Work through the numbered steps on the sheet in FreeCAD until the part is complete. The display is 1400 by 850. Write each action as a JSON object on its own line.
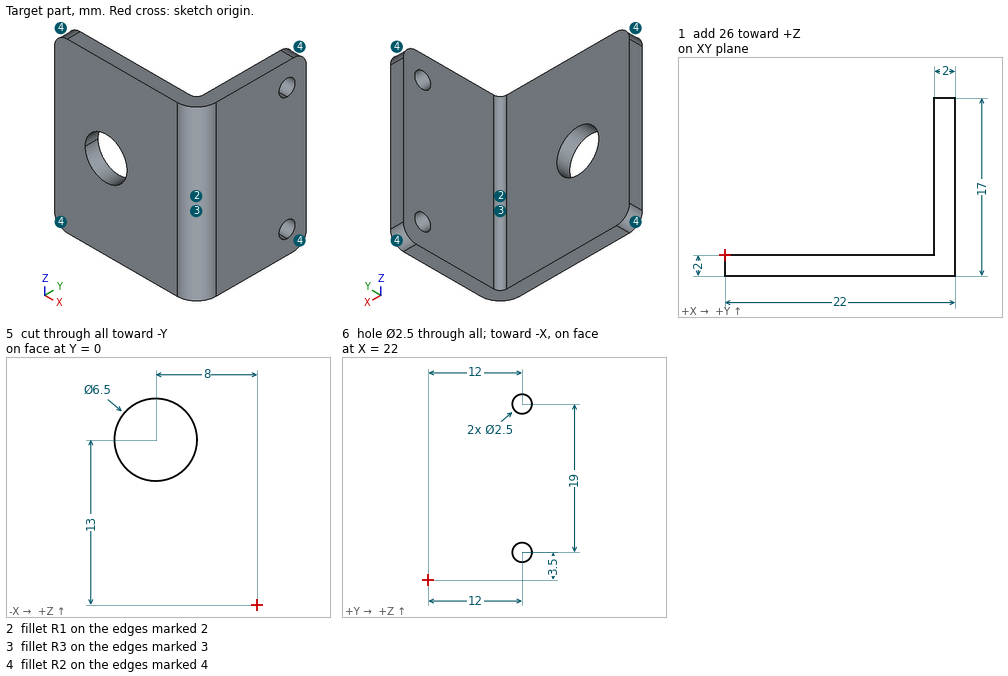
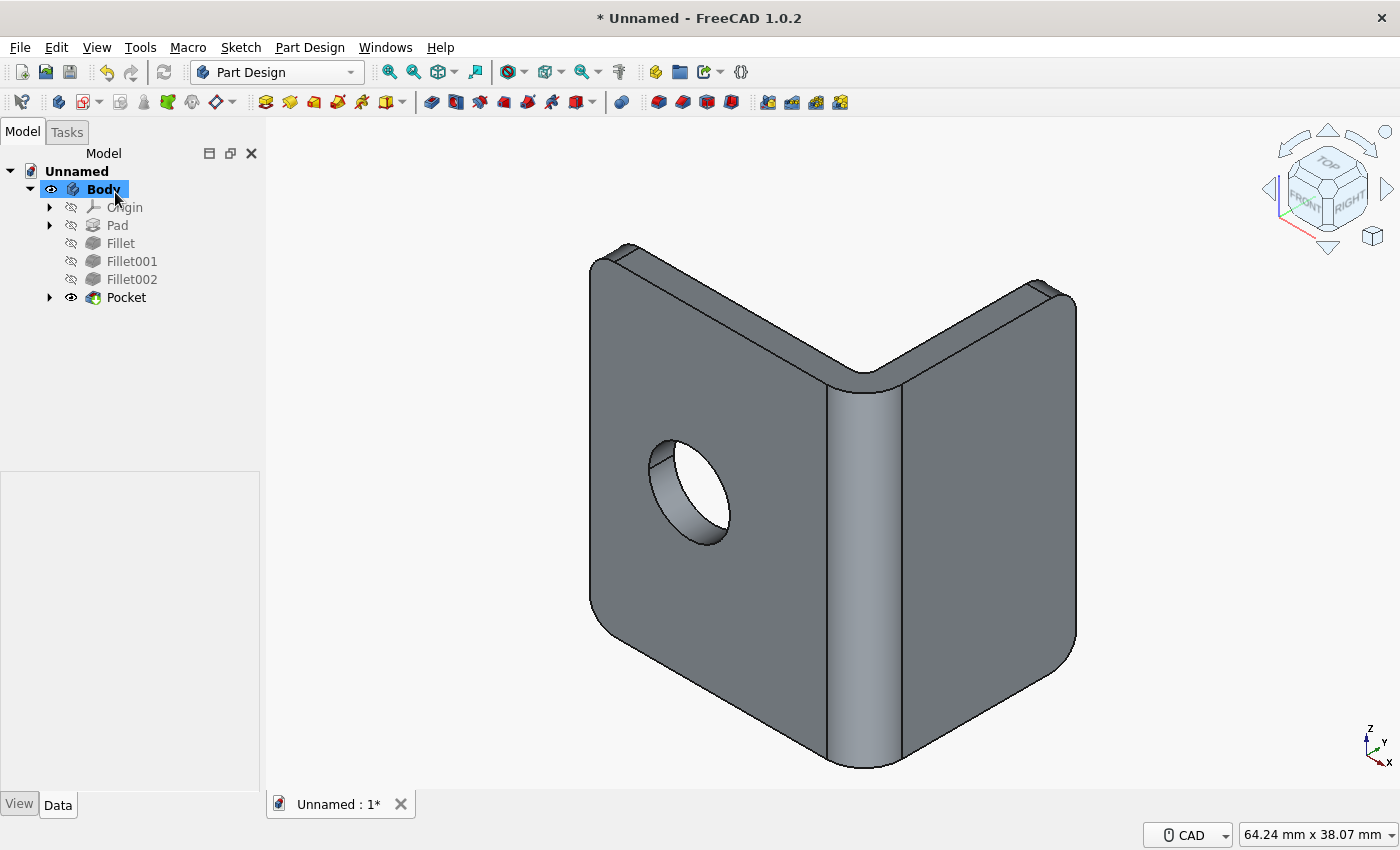
{"action": "left_click", "coordinate": [989, 467]}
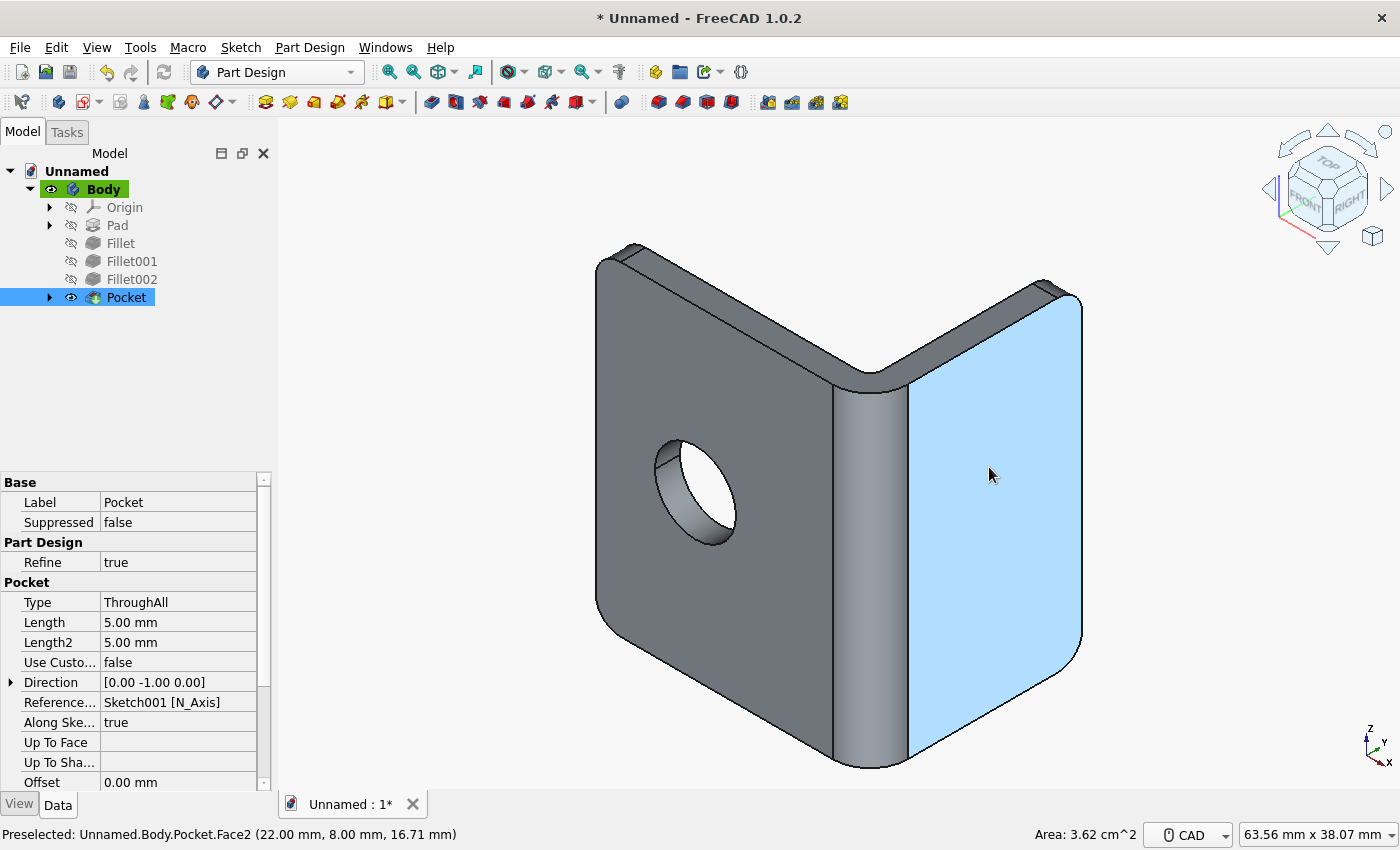
{"action": "left_click", "coordinate": [84, 102]}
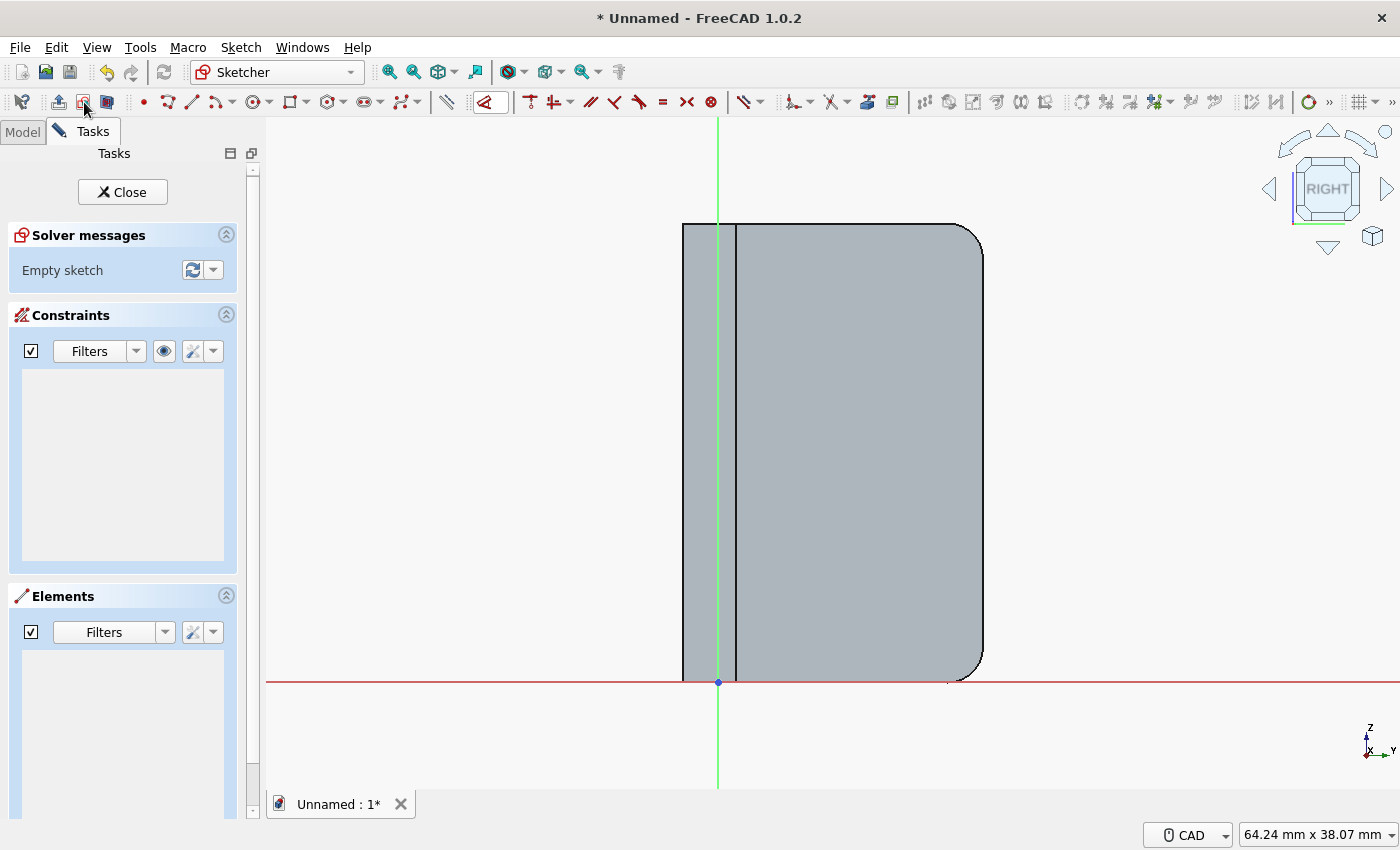
{"action": "key", "text": "g c"}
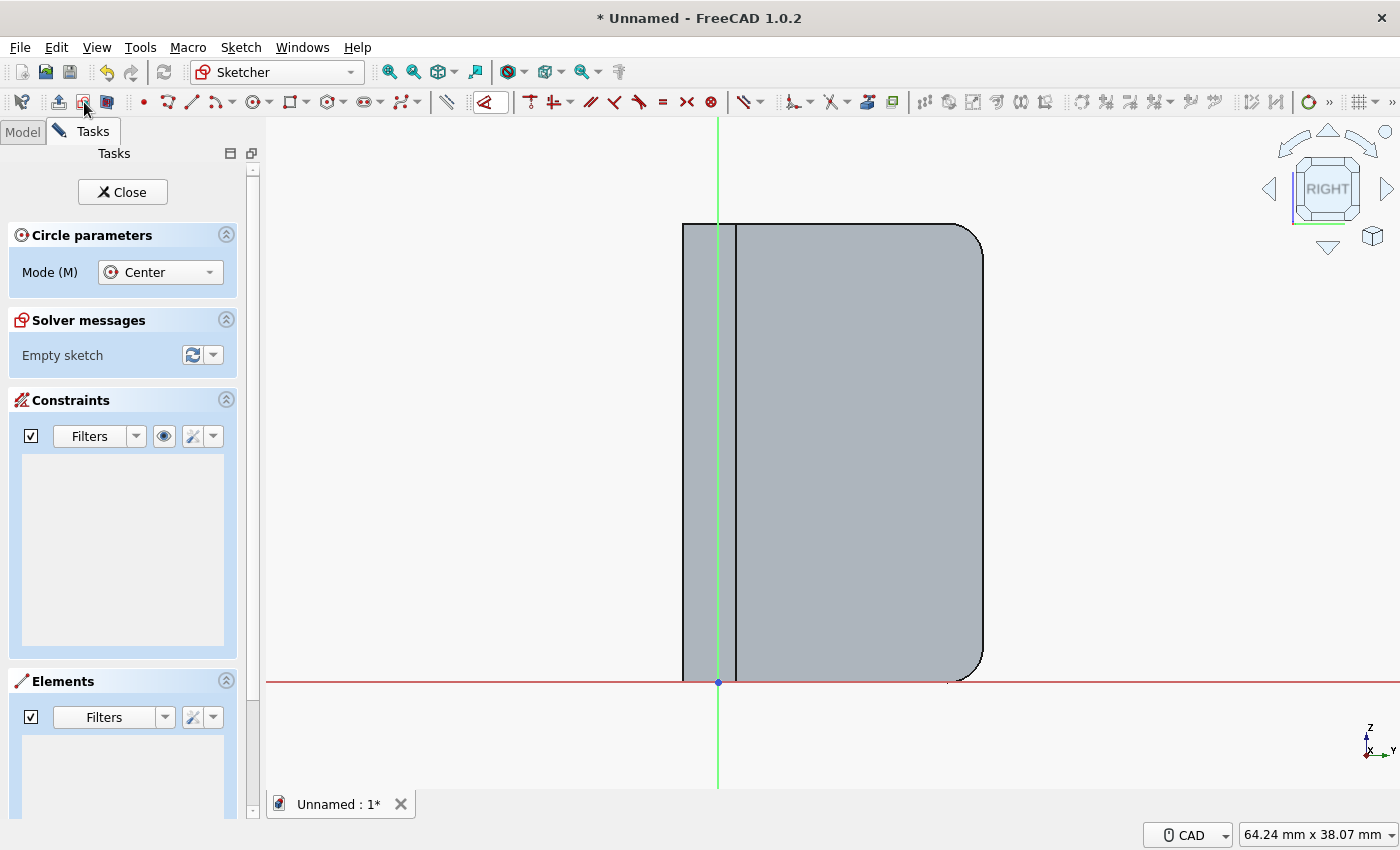
{"action": "left_click", "coordinate": [930, 285]}
{"action": "mouse_move", "coordinate": [946, 270]}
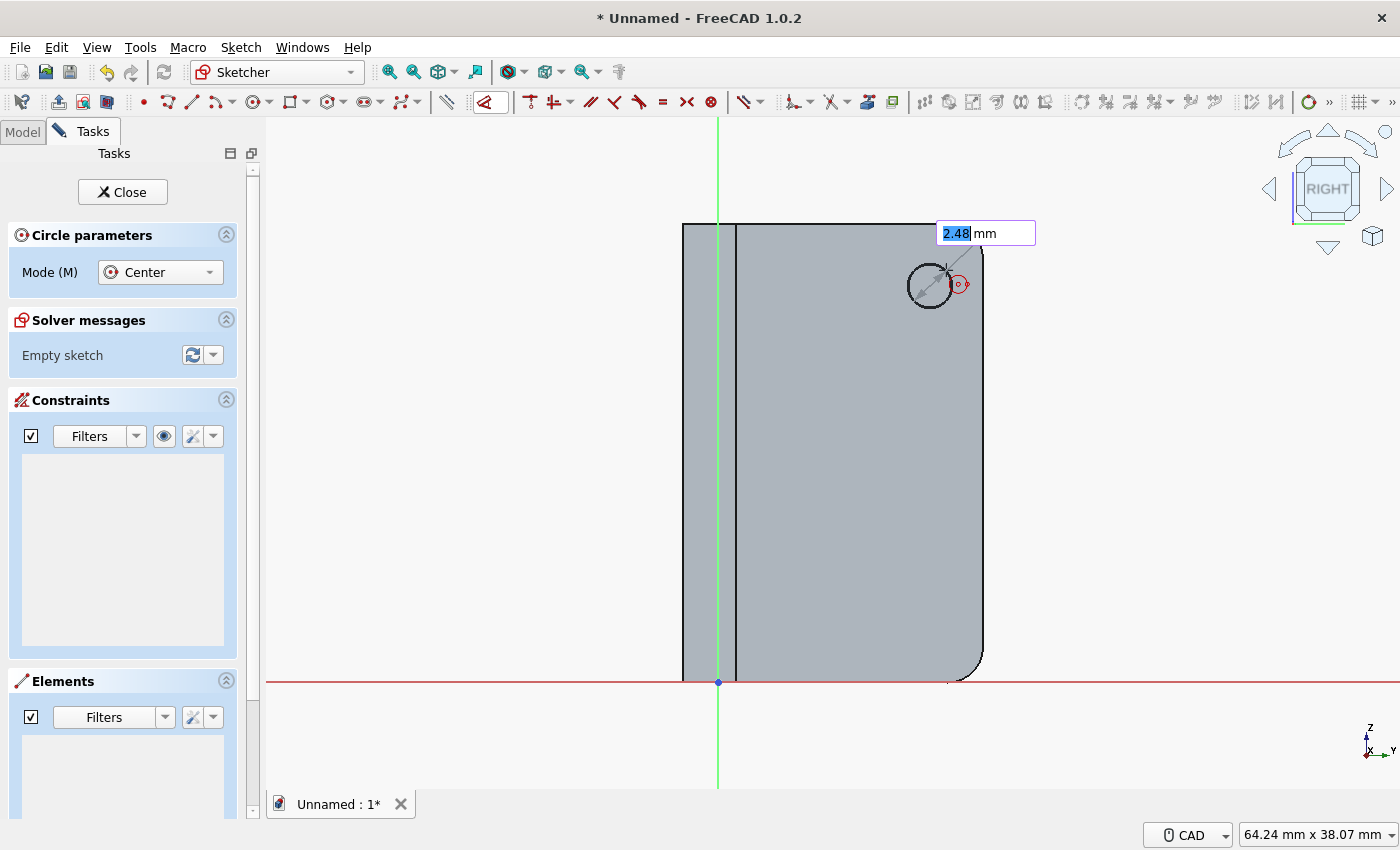
{"action": "type", "text": "2.5"}
{"action": "key", "text": "Return"}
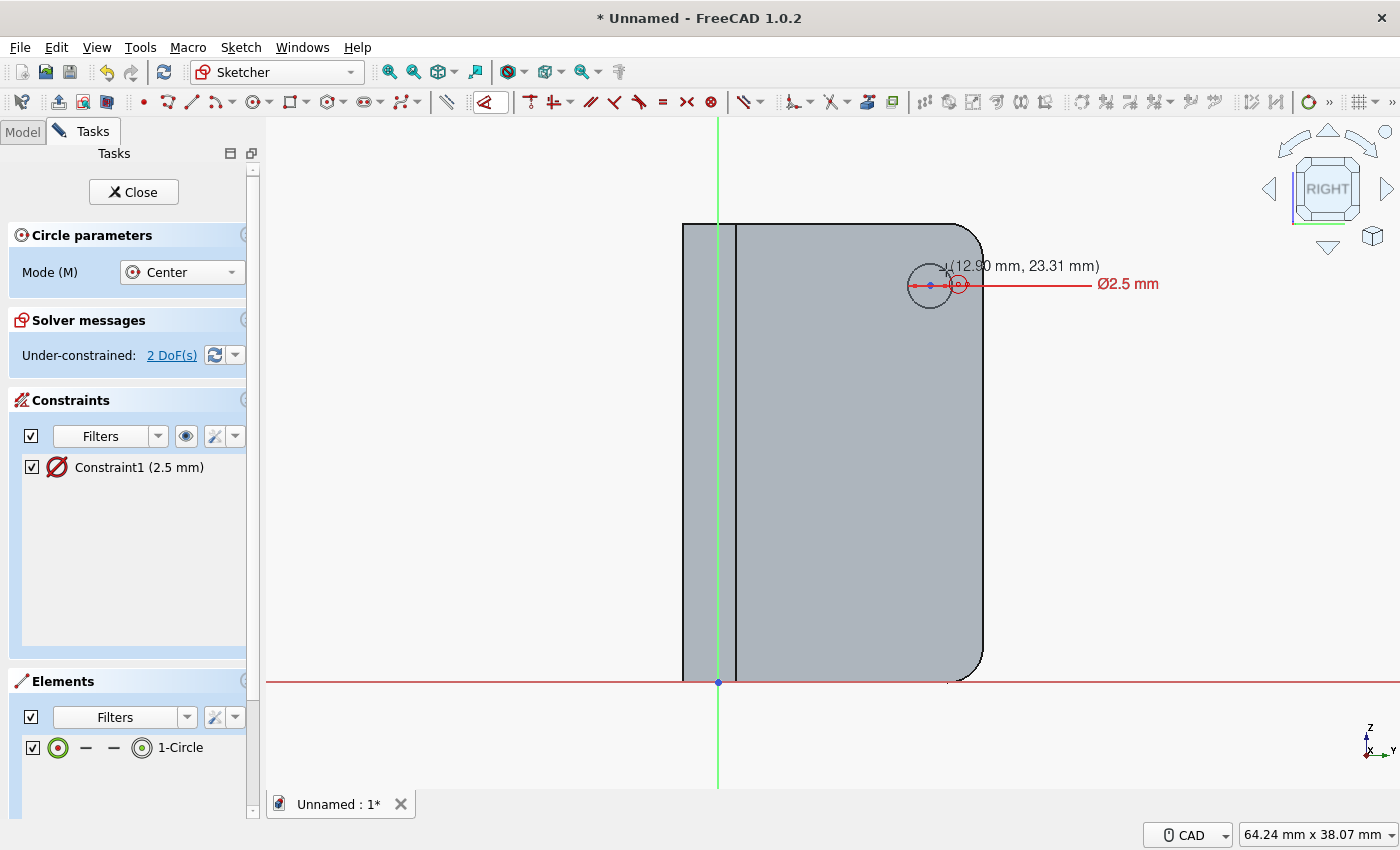
{"action": "left_click", "coordinate": [930, 621]}
{"action": "mouse_move", "coordinate": [946, 605]}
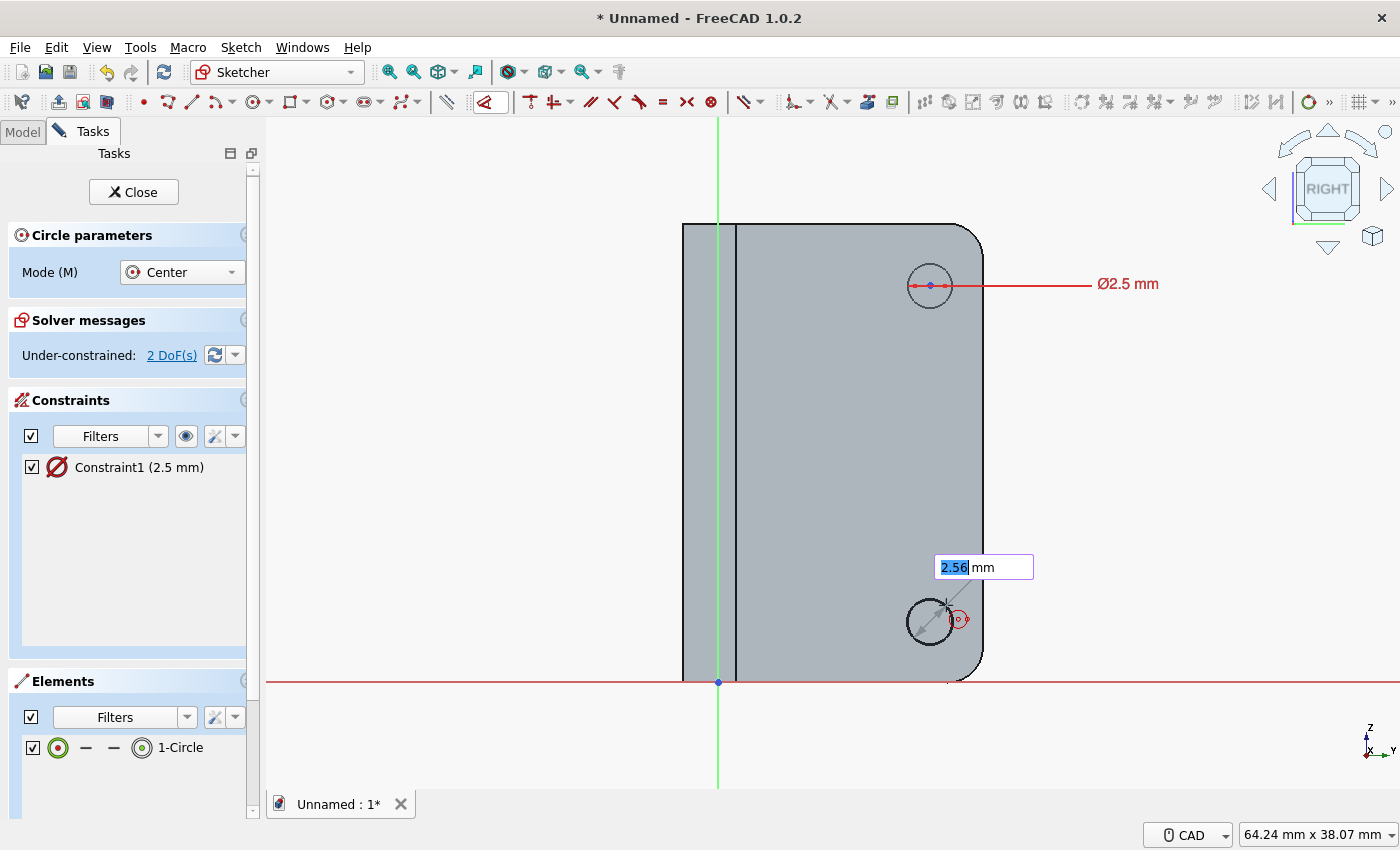
{"action": "type", "text": "2.5"}
{"action": "key", "text": "Return"}
{"action": "key", "text": "Escape"}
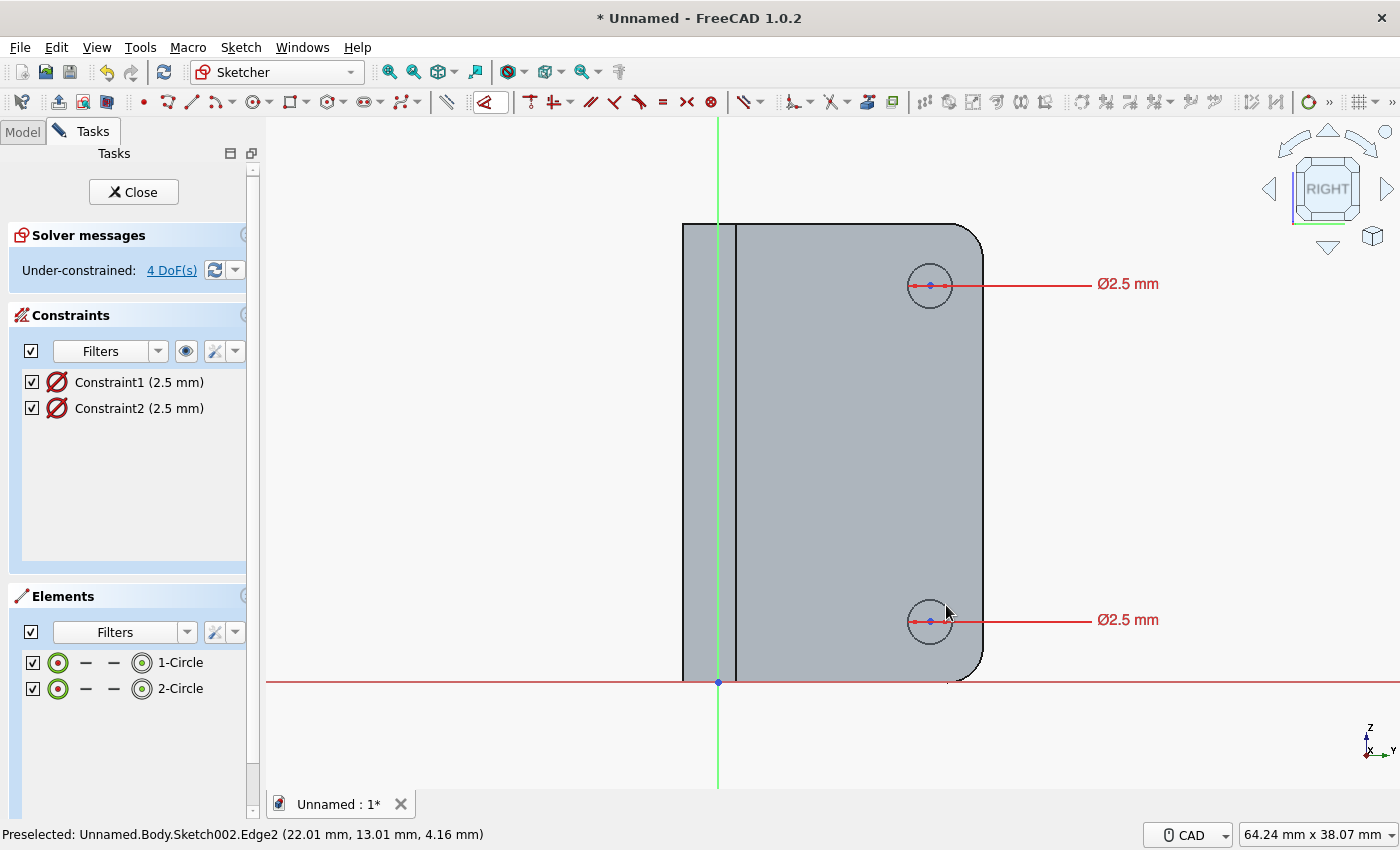
{"action": "left_click", "coordinate": [484, 102]}